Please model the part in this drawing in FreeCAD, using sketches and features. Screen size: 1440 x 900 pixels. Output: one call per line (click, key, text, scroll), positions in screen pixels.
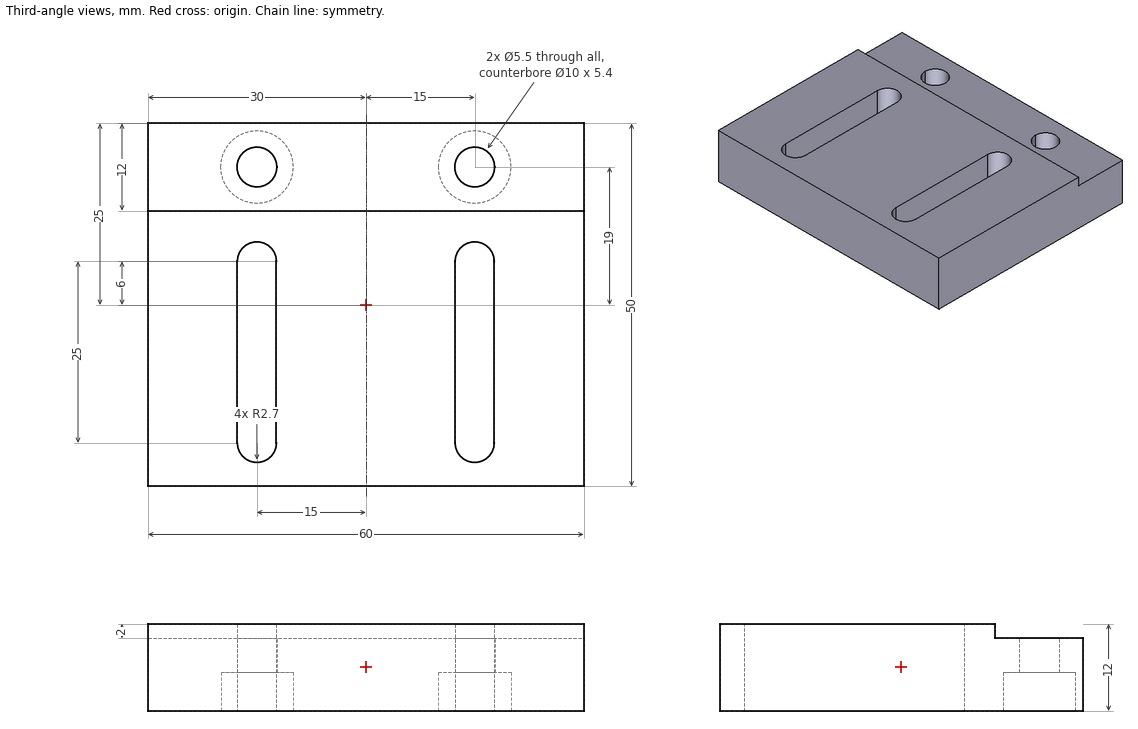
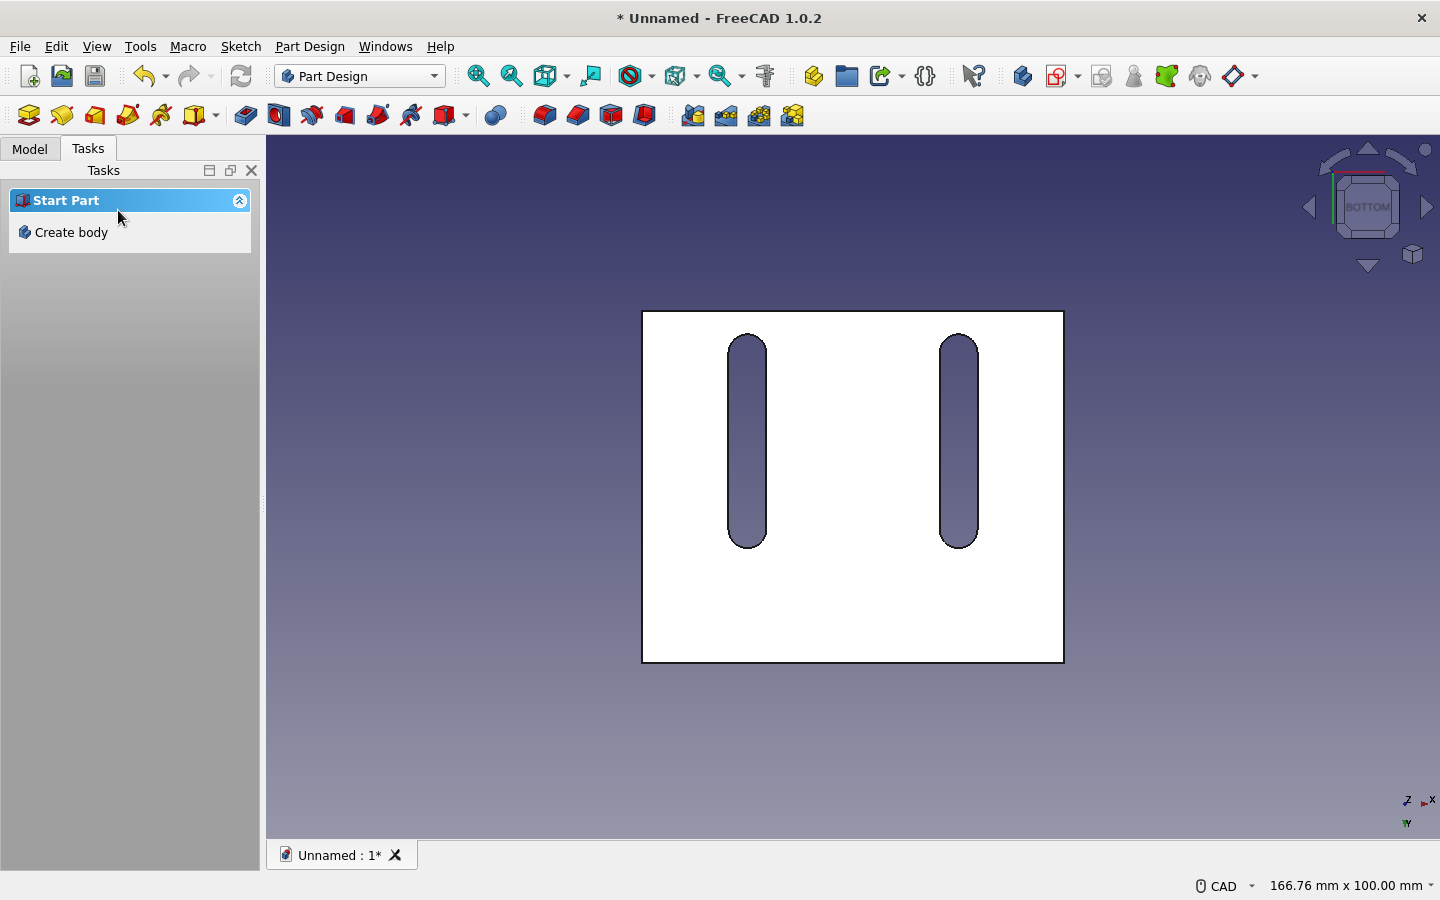
click(853, 536)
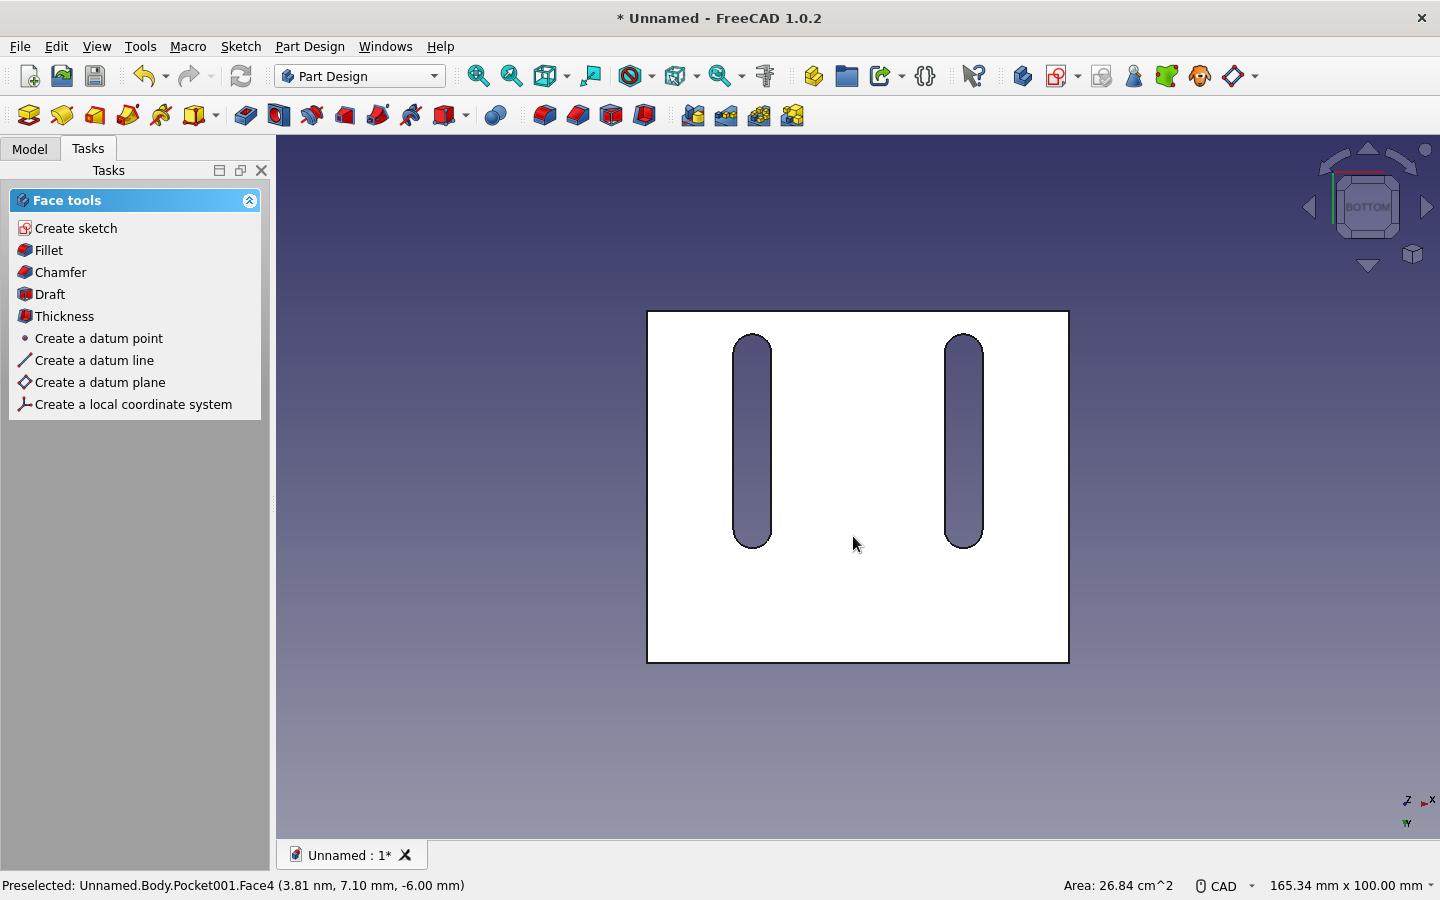
click(1056, 76)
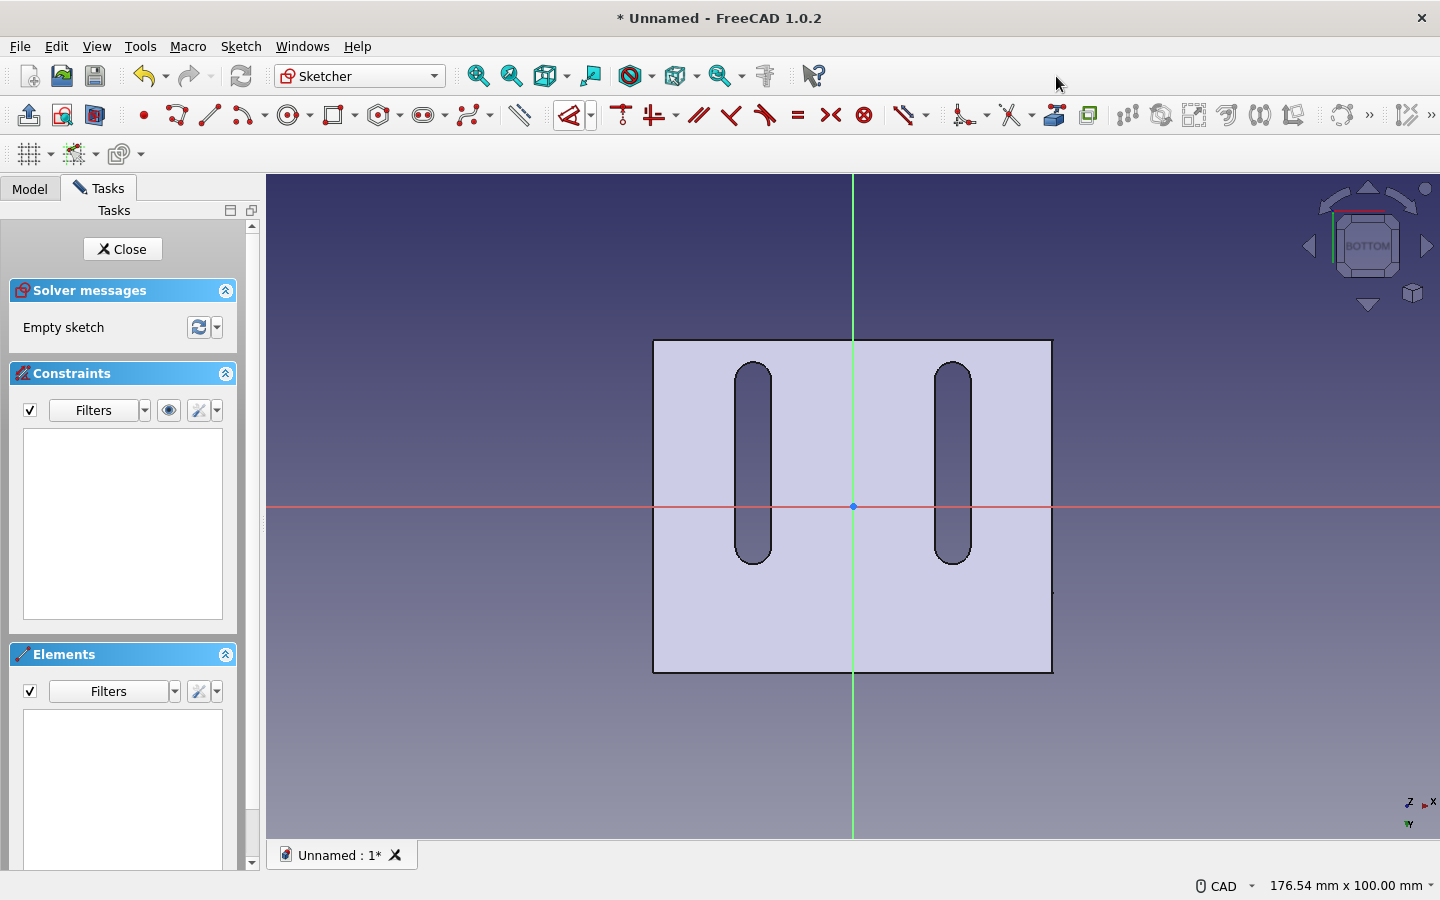
scroll(893, 621, up, 5)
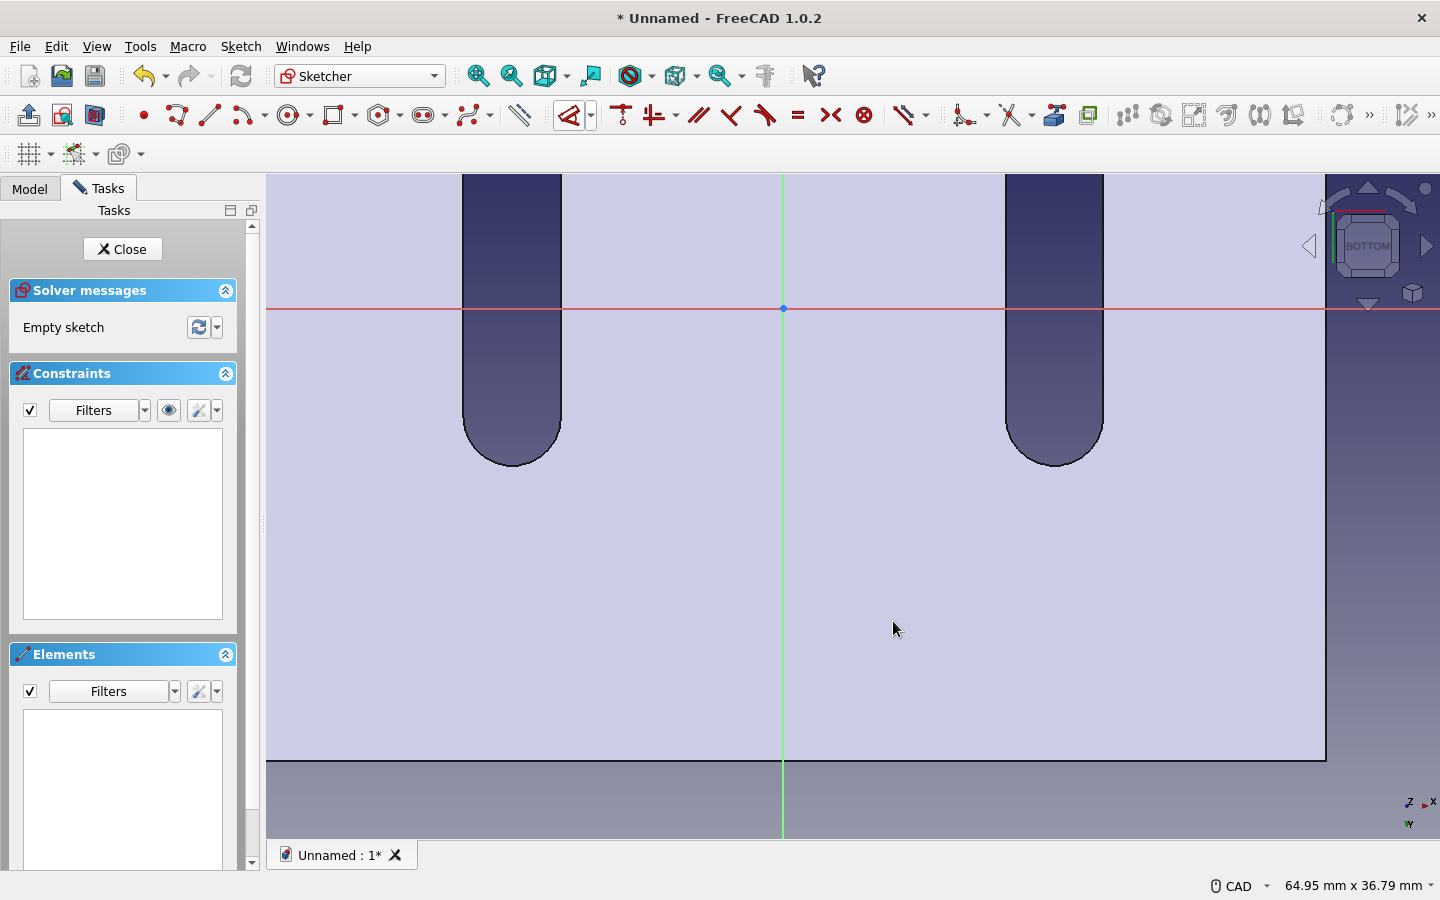
click(288, 116)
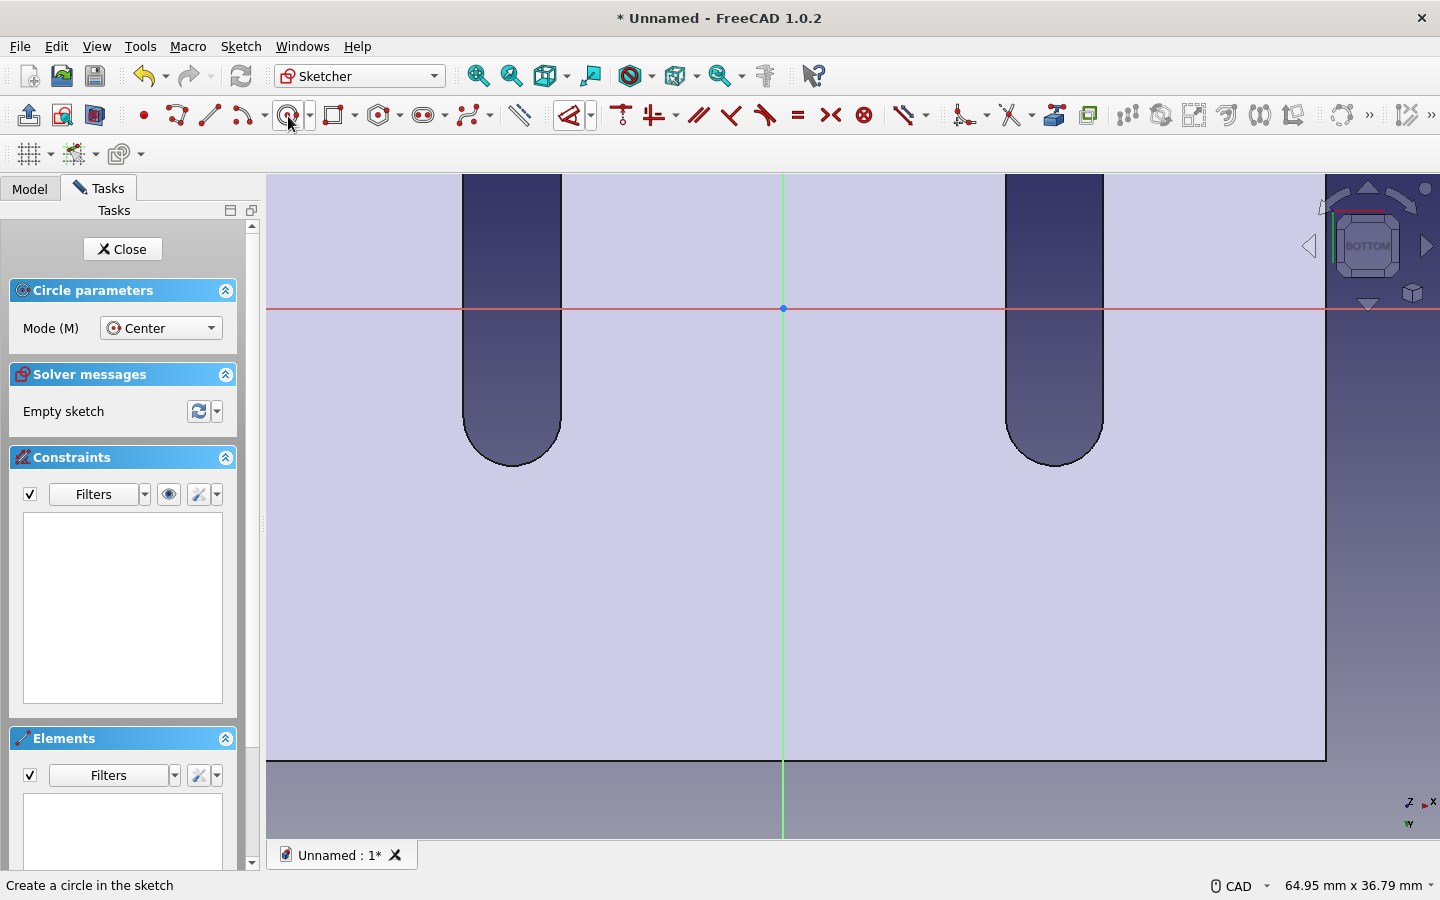
click(1054, 652)
click(1090, 617)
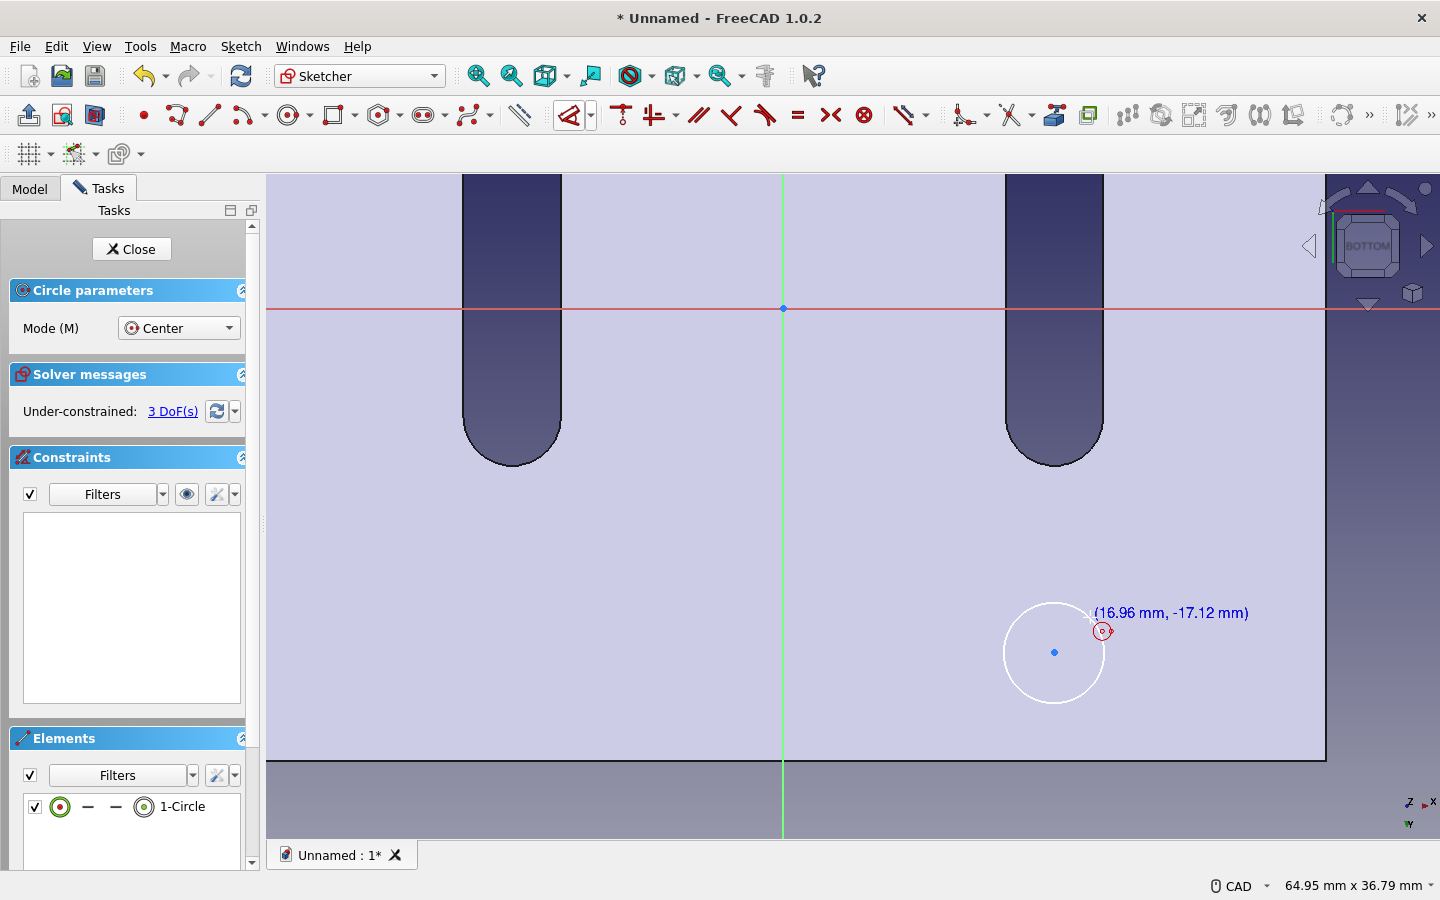
click(512, 652)
click(547, 617)
key(Escape)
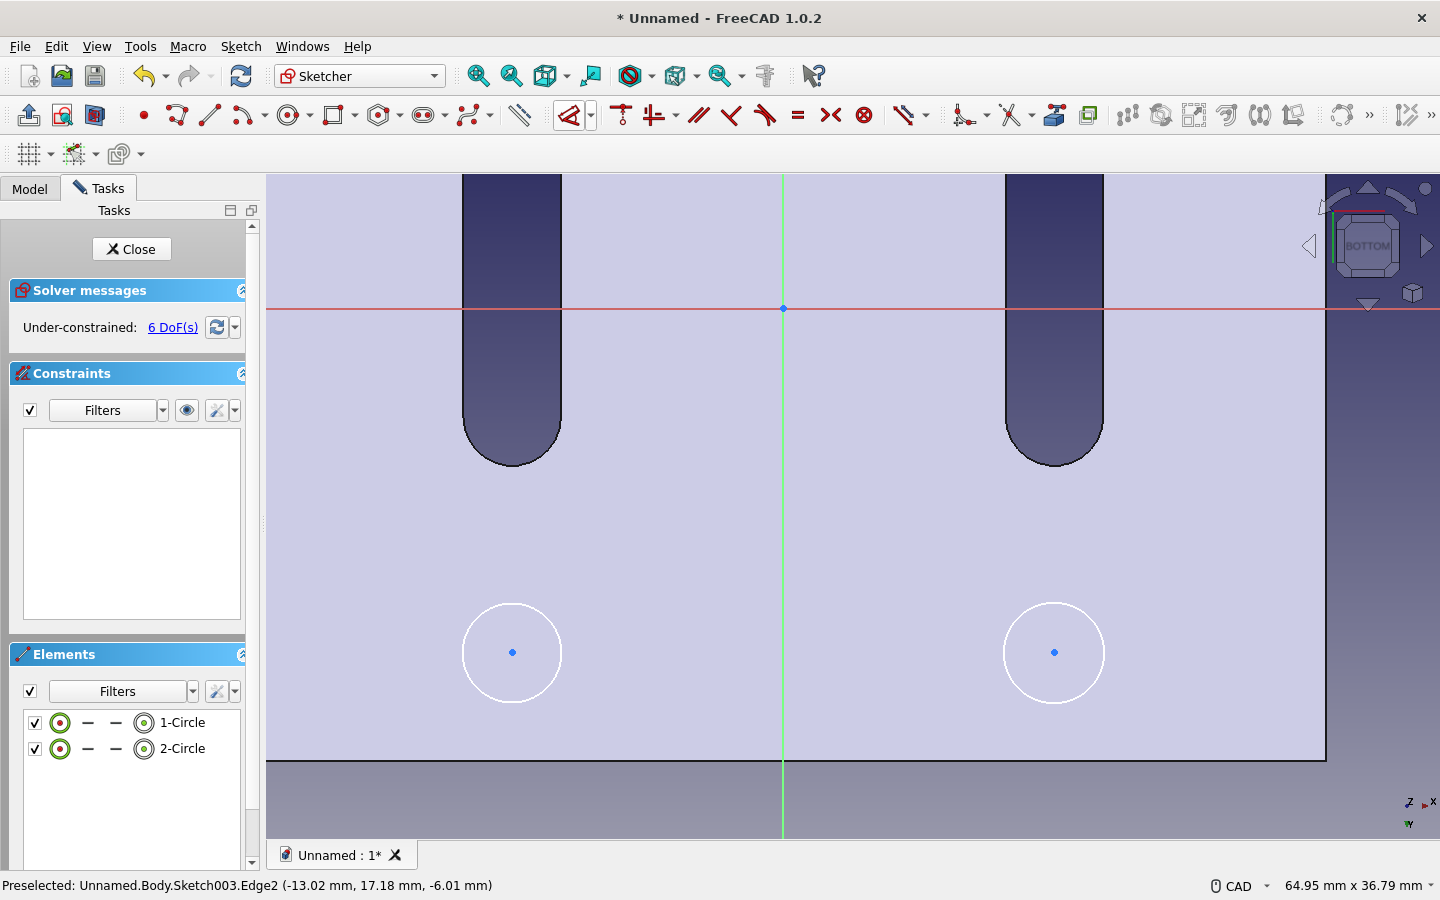
click(1089, 617)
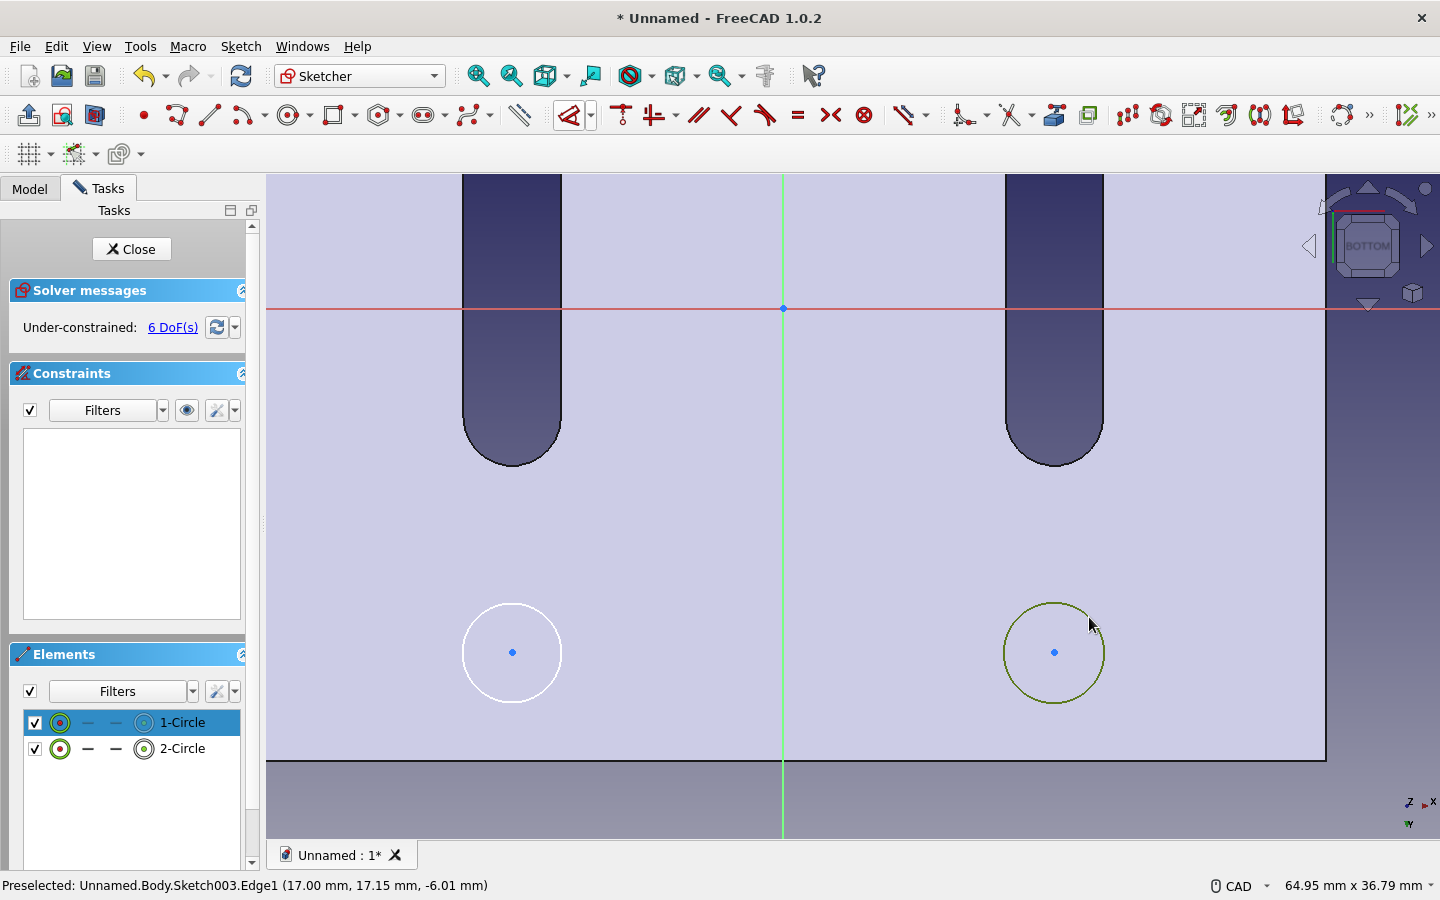
click(547, 618)